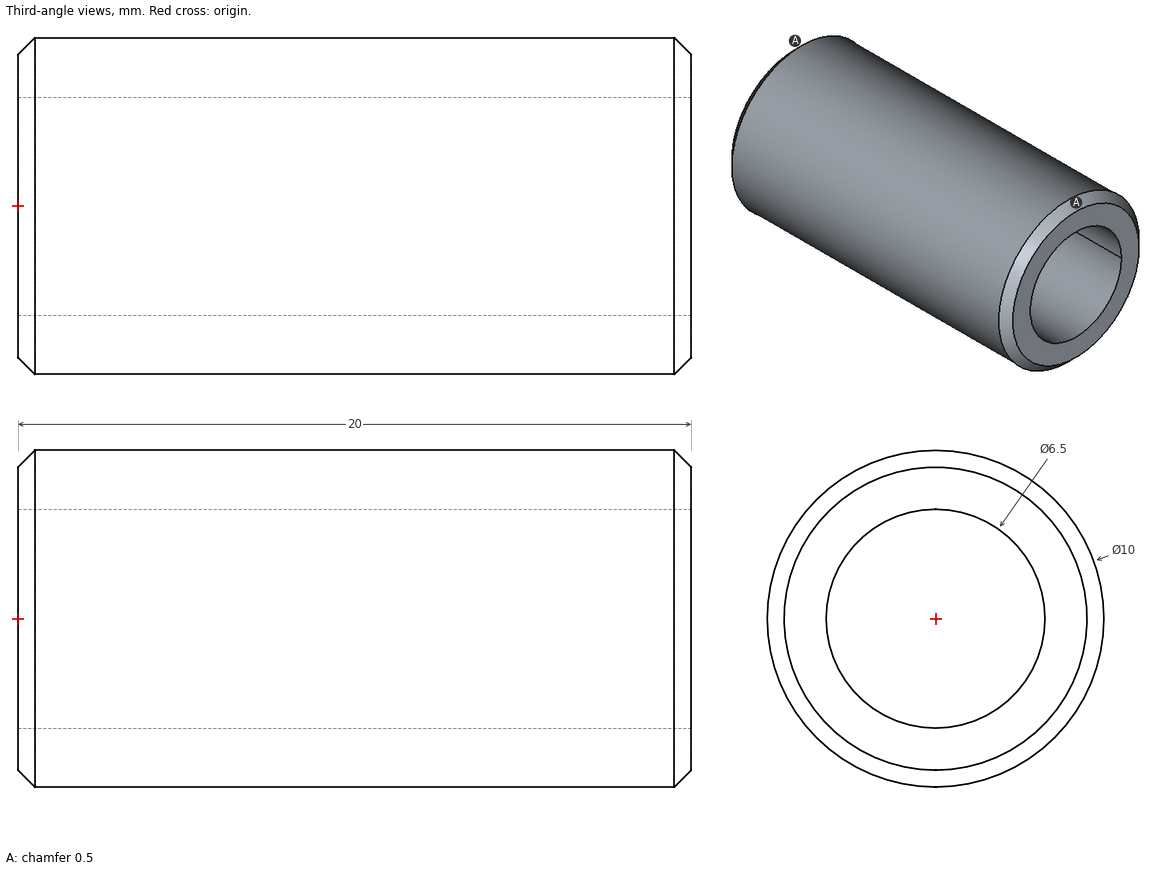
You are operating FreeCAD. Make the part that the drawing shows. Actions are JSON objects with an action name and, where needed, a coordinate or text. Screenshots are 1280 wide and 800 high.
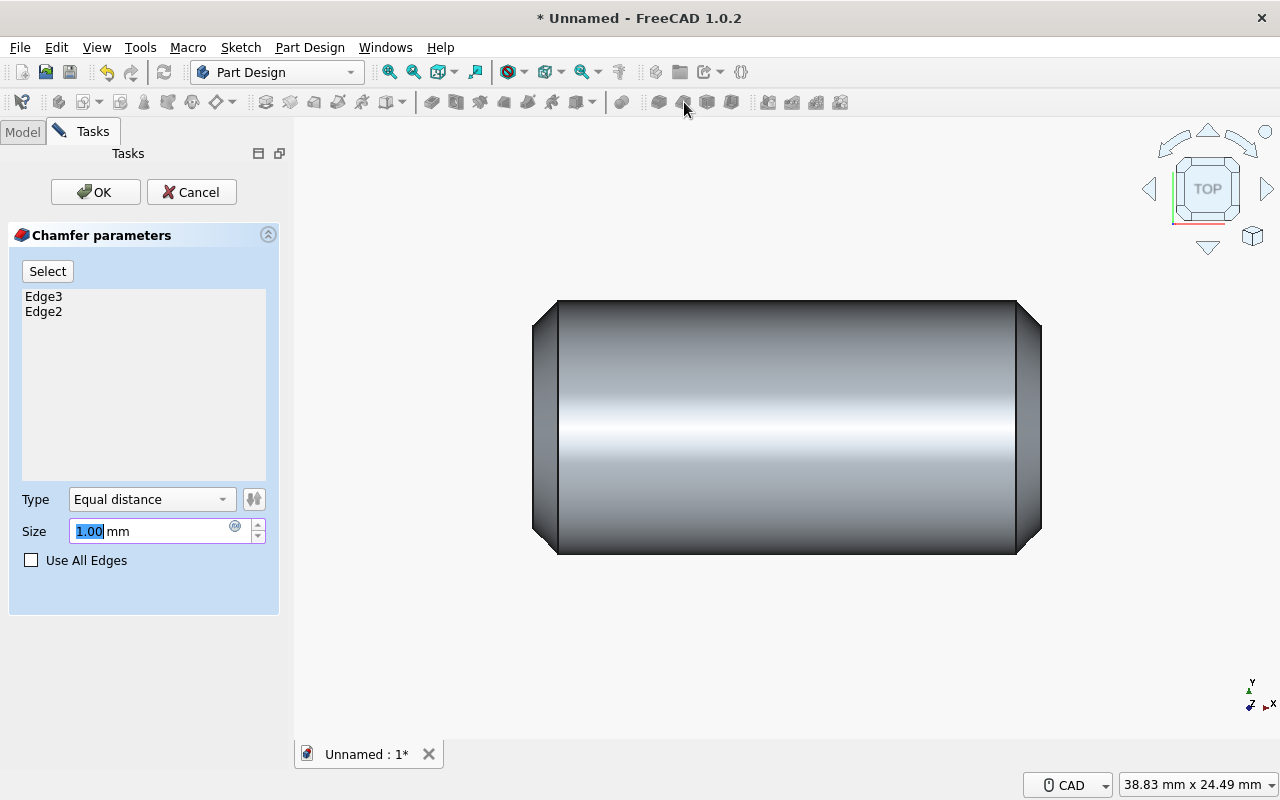
{"action": "type", "text": "0.5"}
{"action": "key", "text": "Tab"}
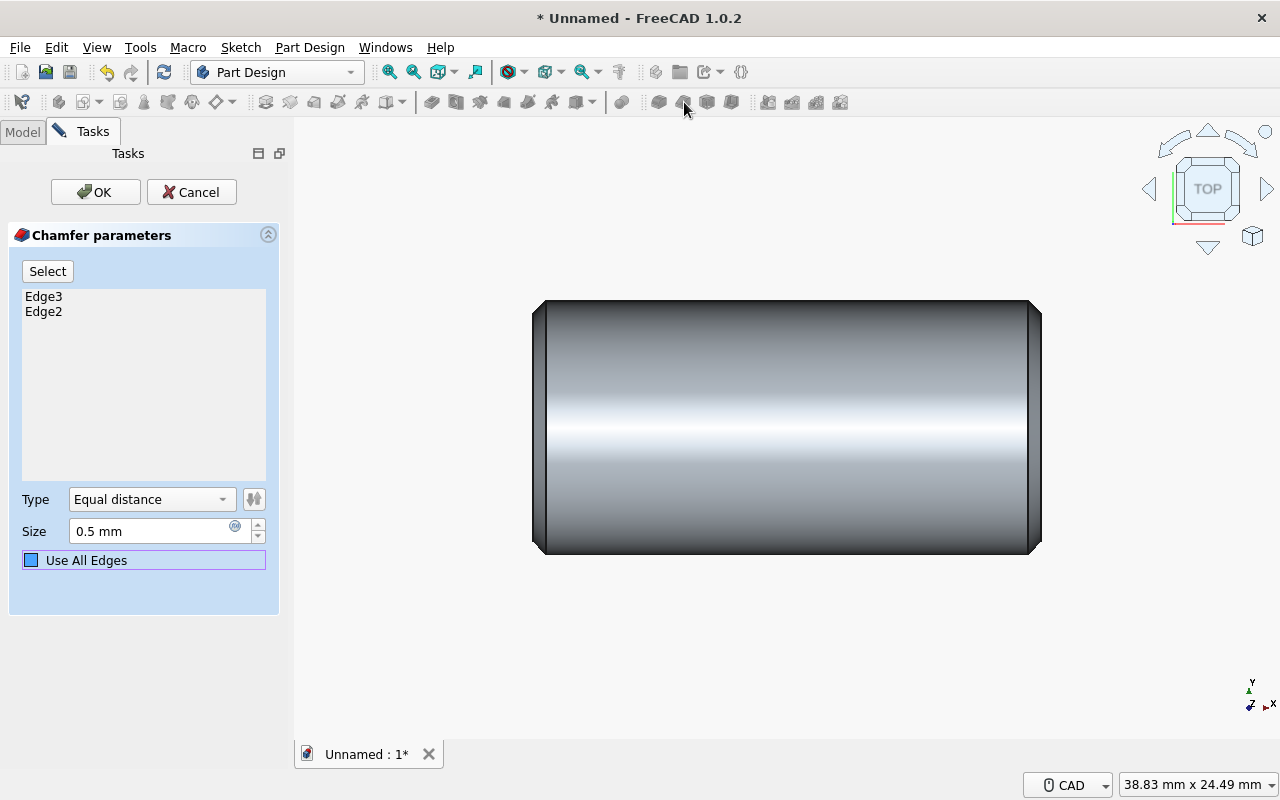
{"action": "left_click", "coordinate": [96, 192]}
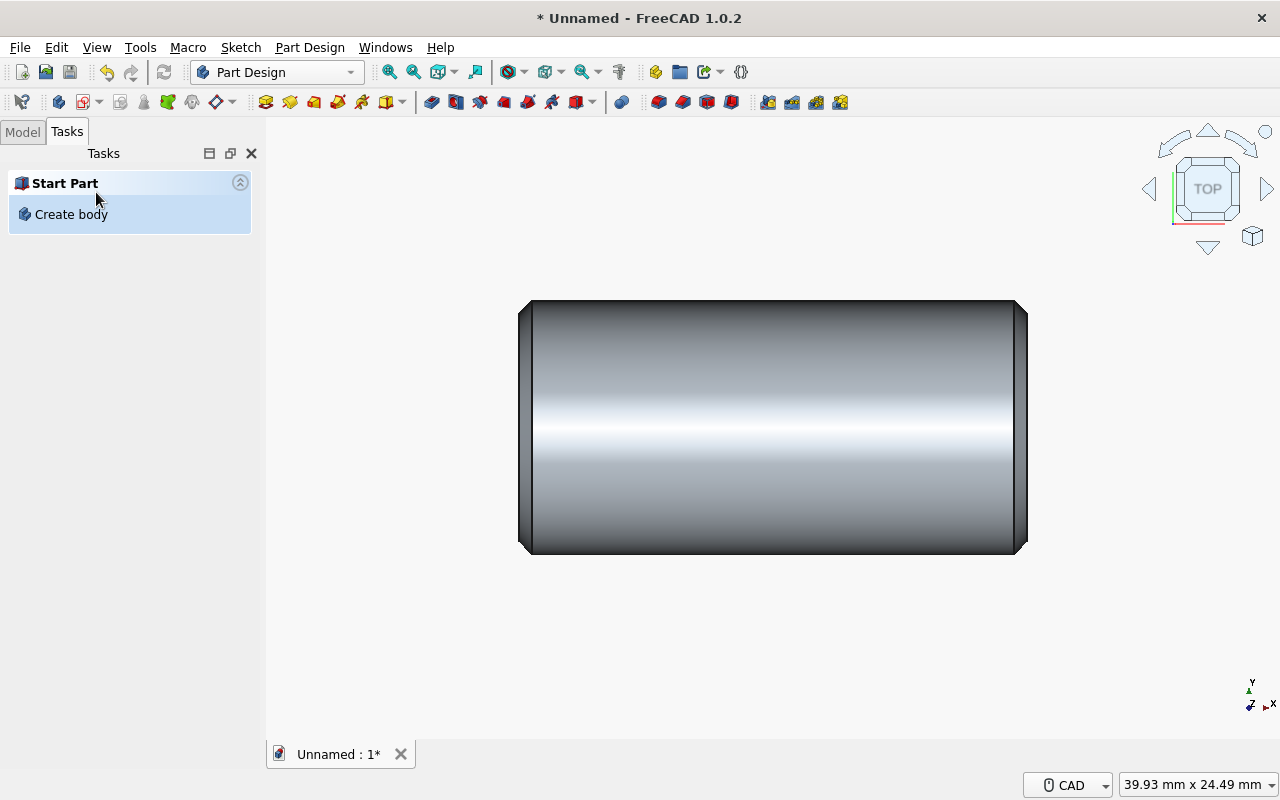
{"action": "left_click", "coordinate": [84, 102]}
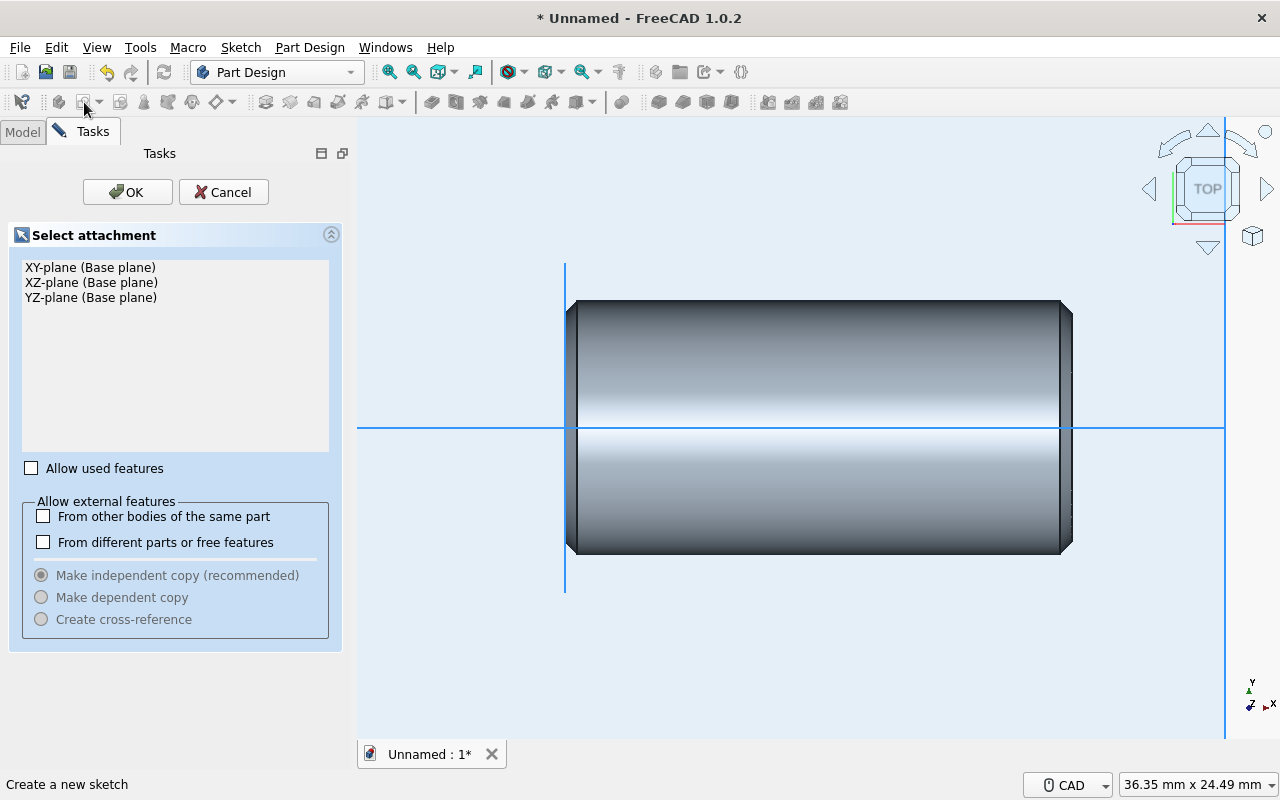
{"action": "left_click", "coordinate": [82, 298]}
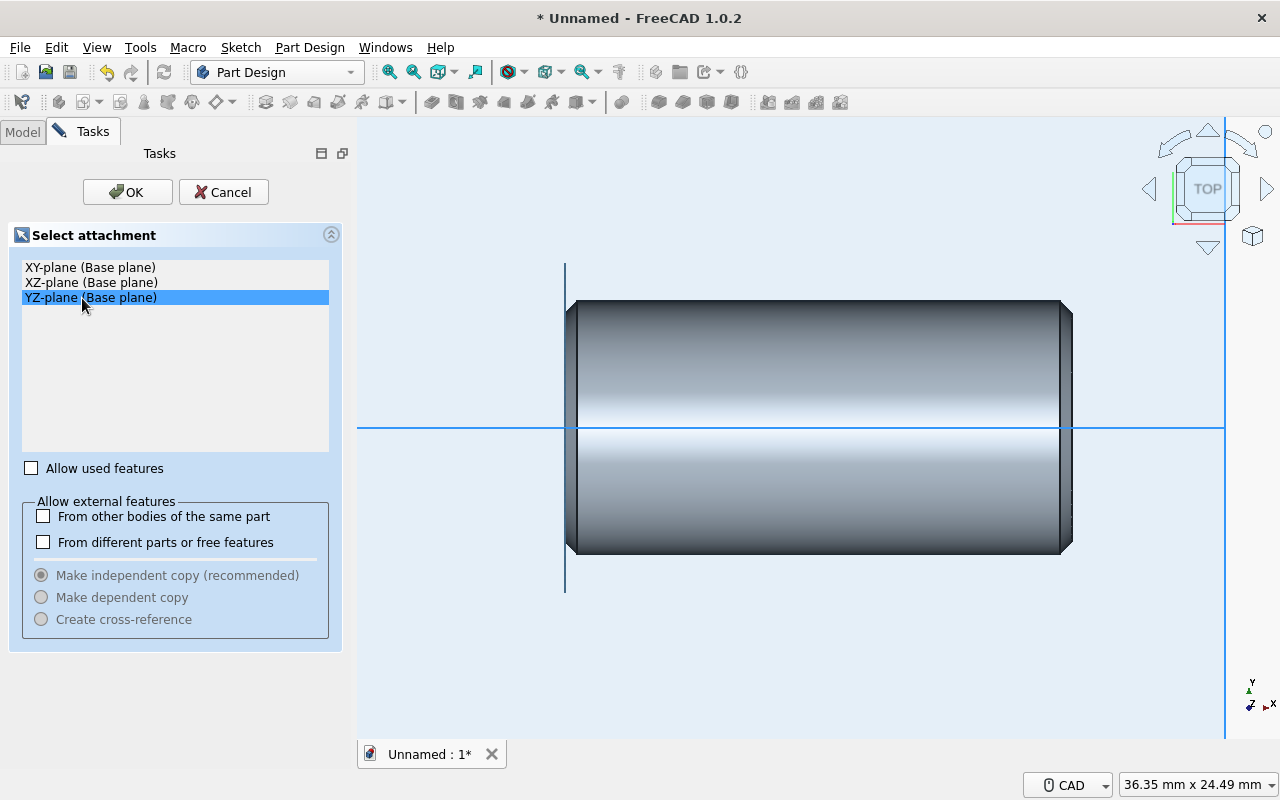
{"action": "left_click", "coordinate": [128, 192]}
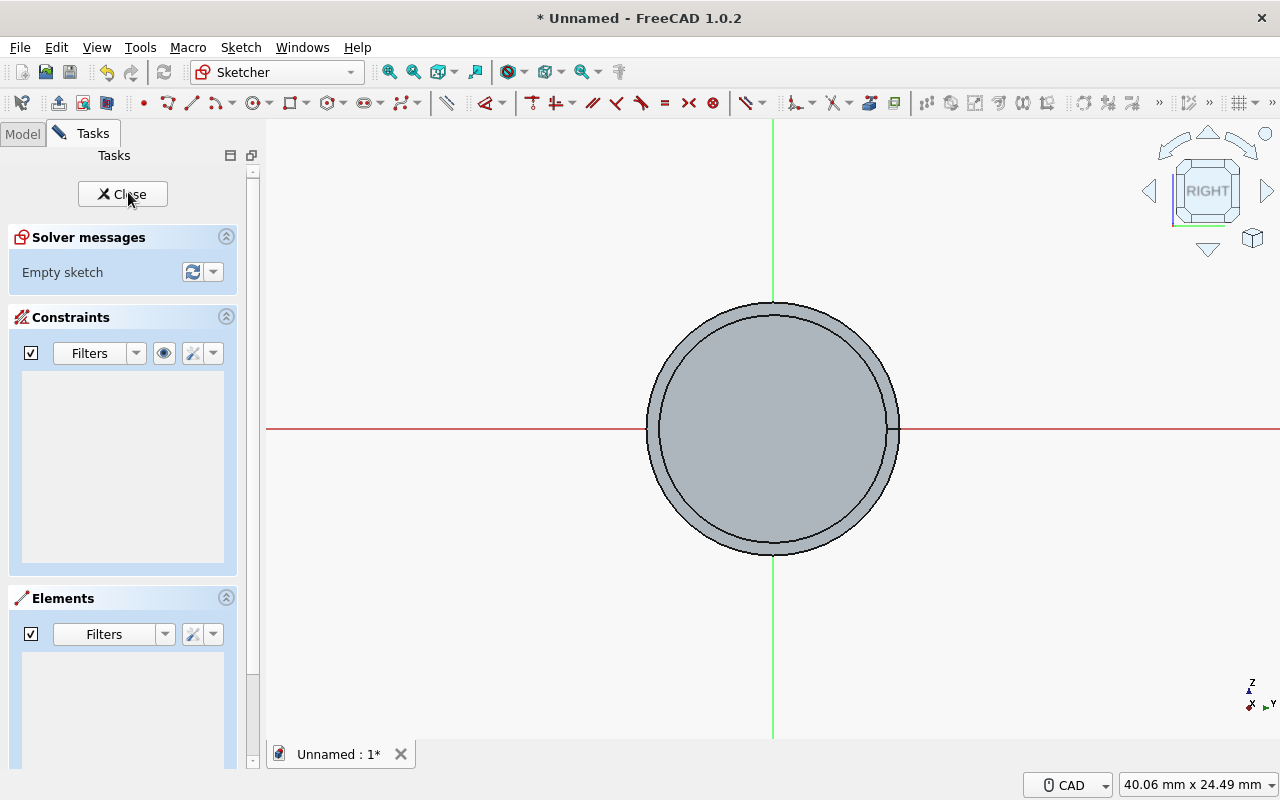
{"action": "key", "text": "q s"}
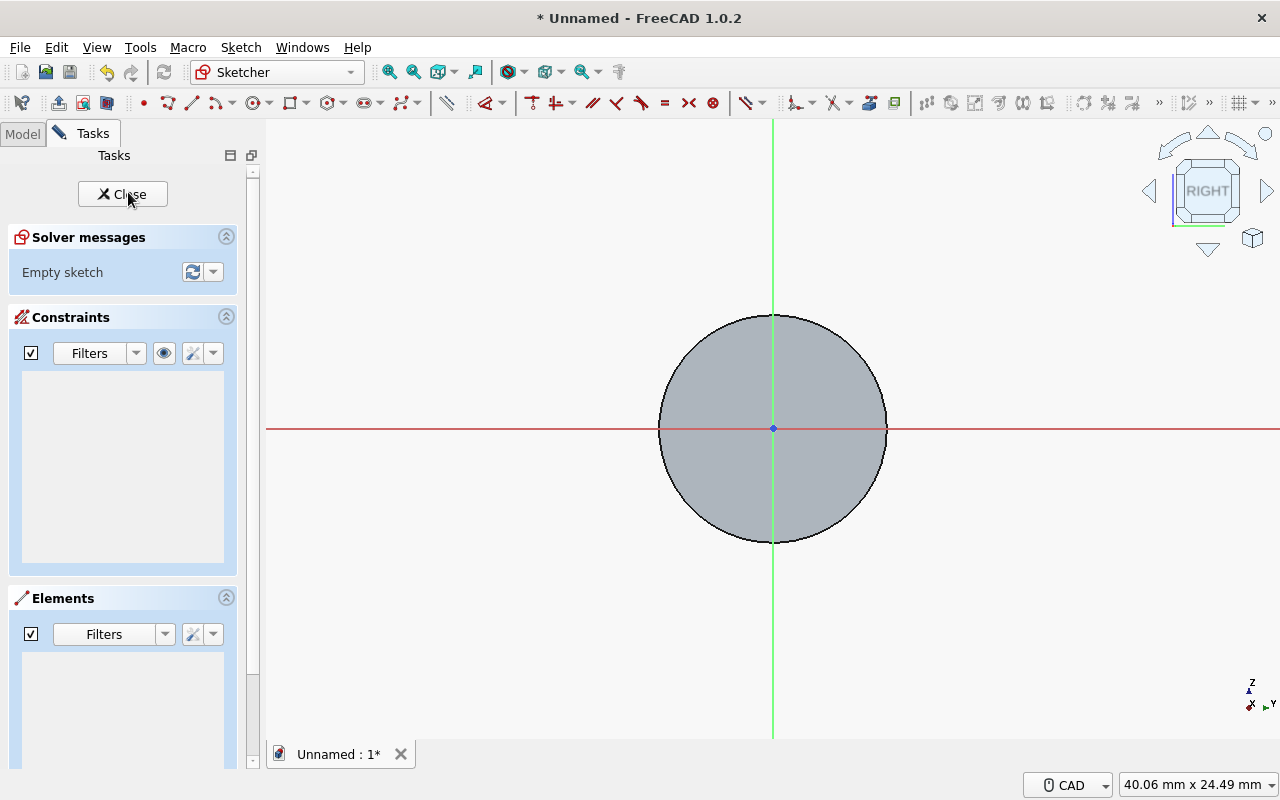
{"action": "scroll", "coordinate": [829, 429], "scroll_direction": "up", "scroll_amount": 4}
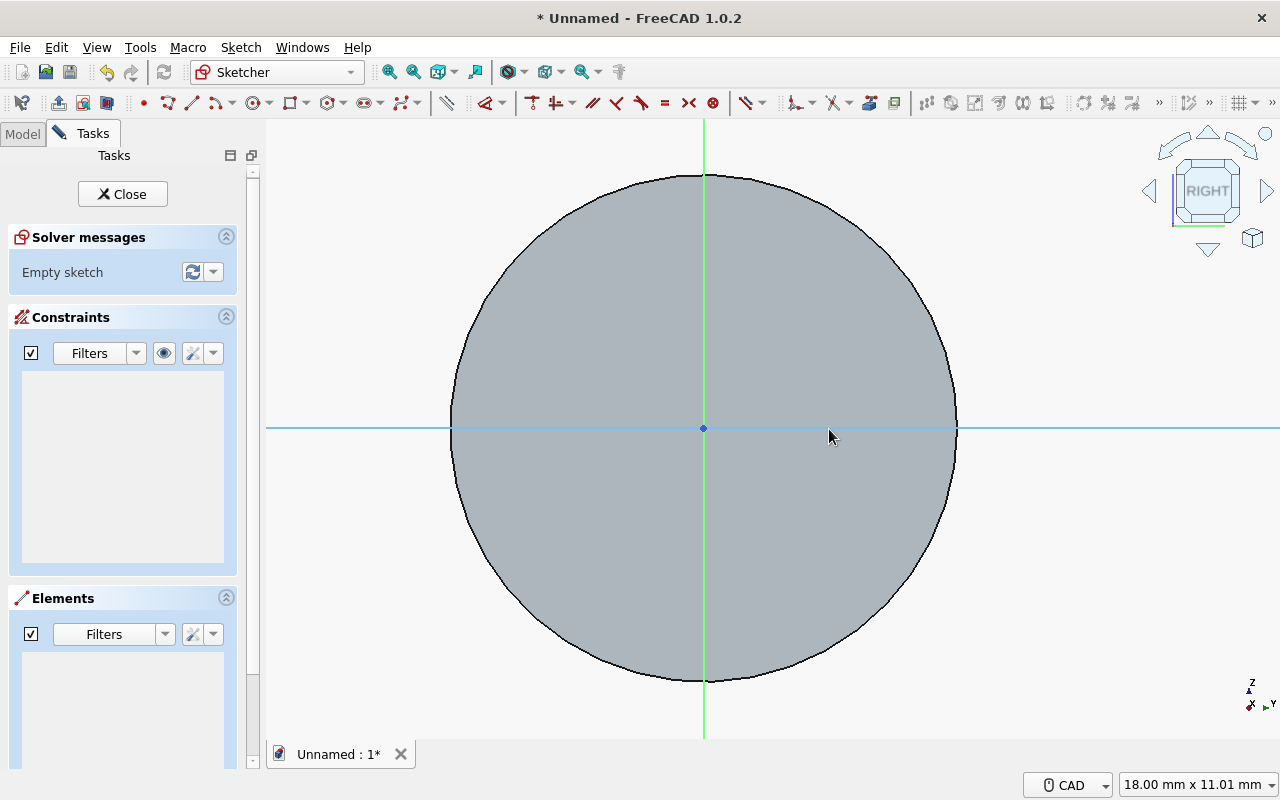
{"action": "left_click", "coordinate": [254, 104]}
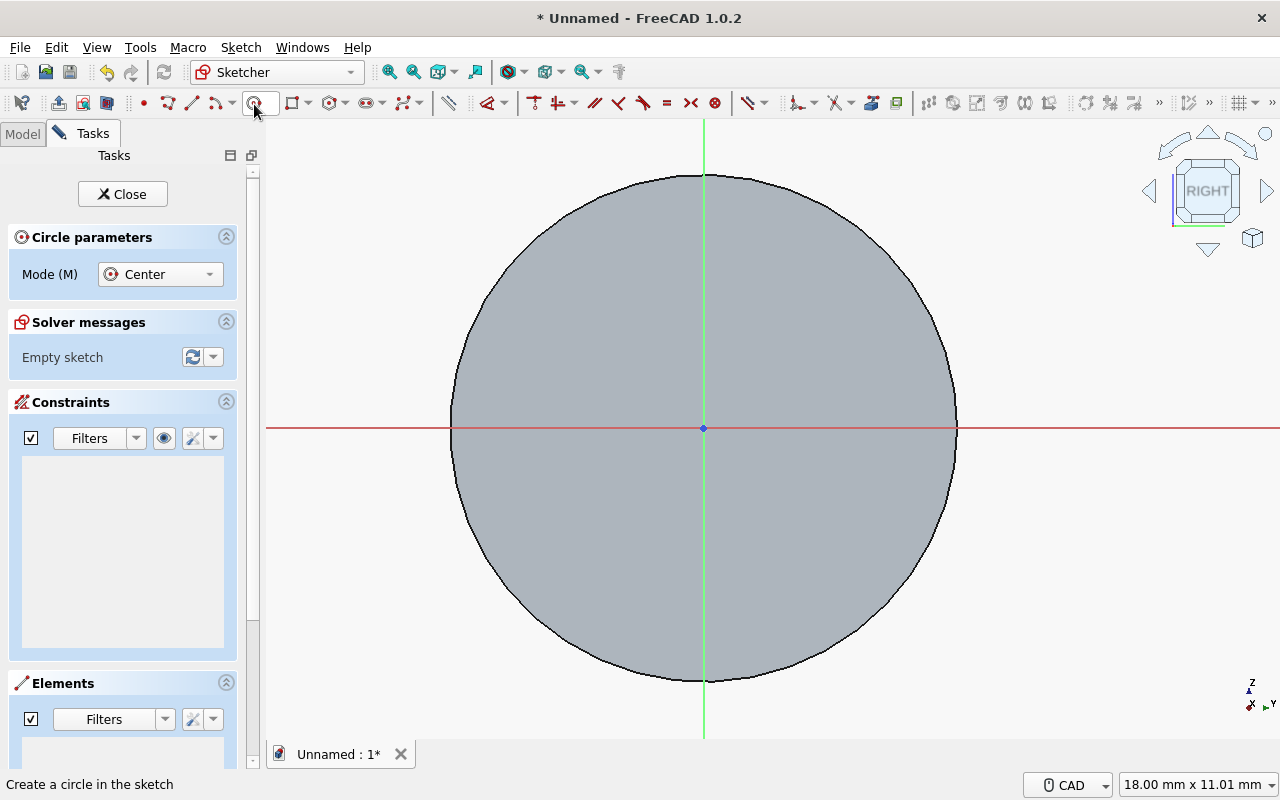
{"action": "left_click", "coordinate": [704, 428]}
{"action": "left_click", "coordinate": [833, 299]}
{"action": "key", "text": "Escape"}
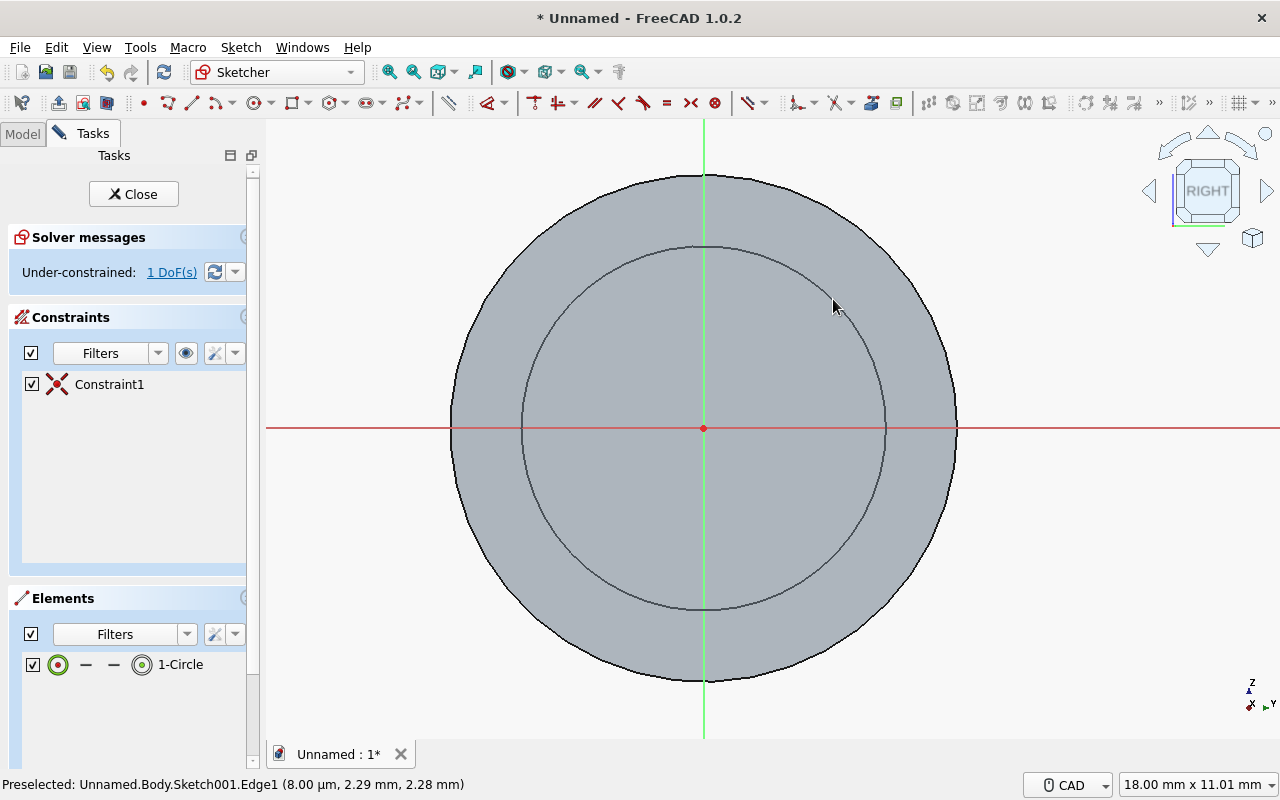
{"action": "left_click", "coordinate": [488, 104]}